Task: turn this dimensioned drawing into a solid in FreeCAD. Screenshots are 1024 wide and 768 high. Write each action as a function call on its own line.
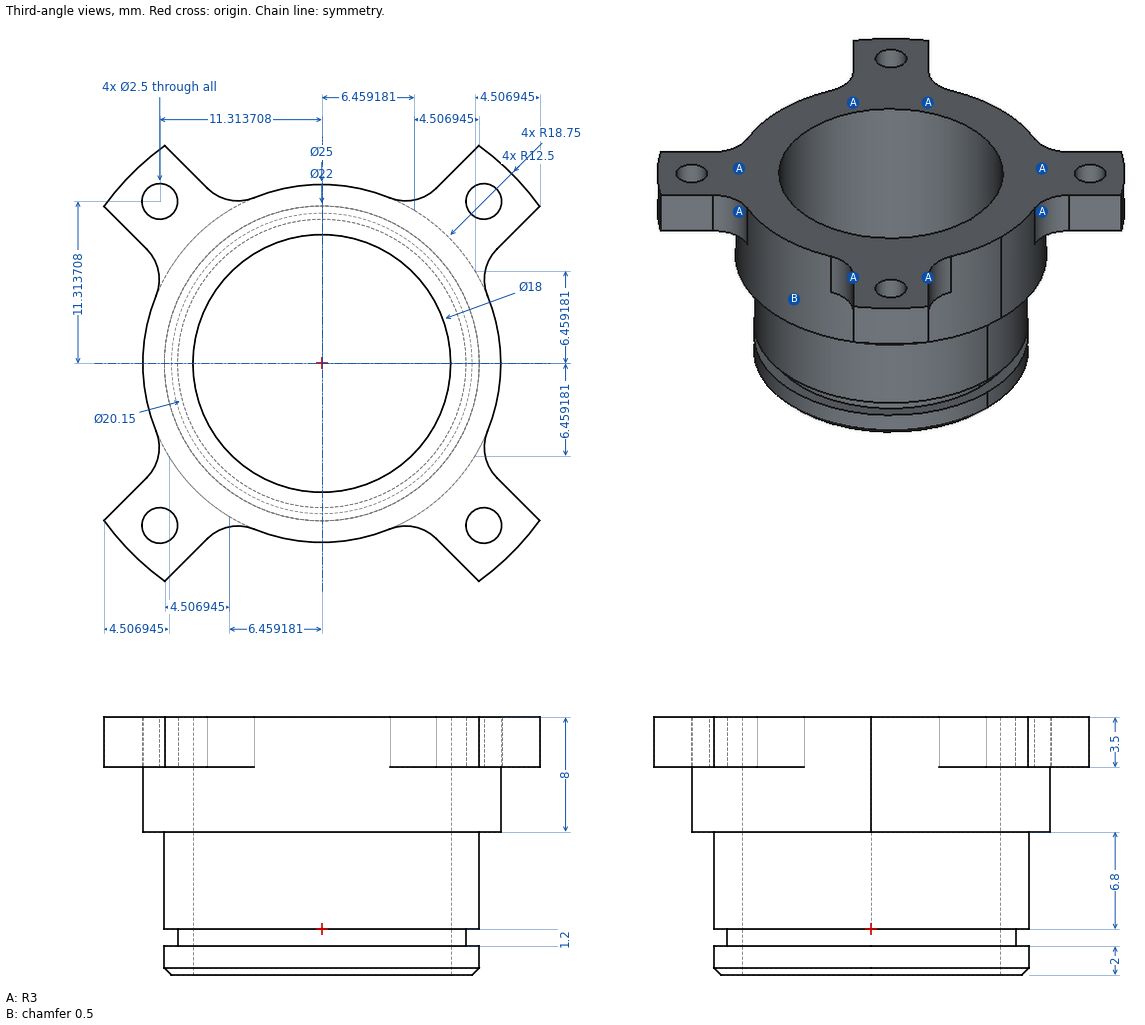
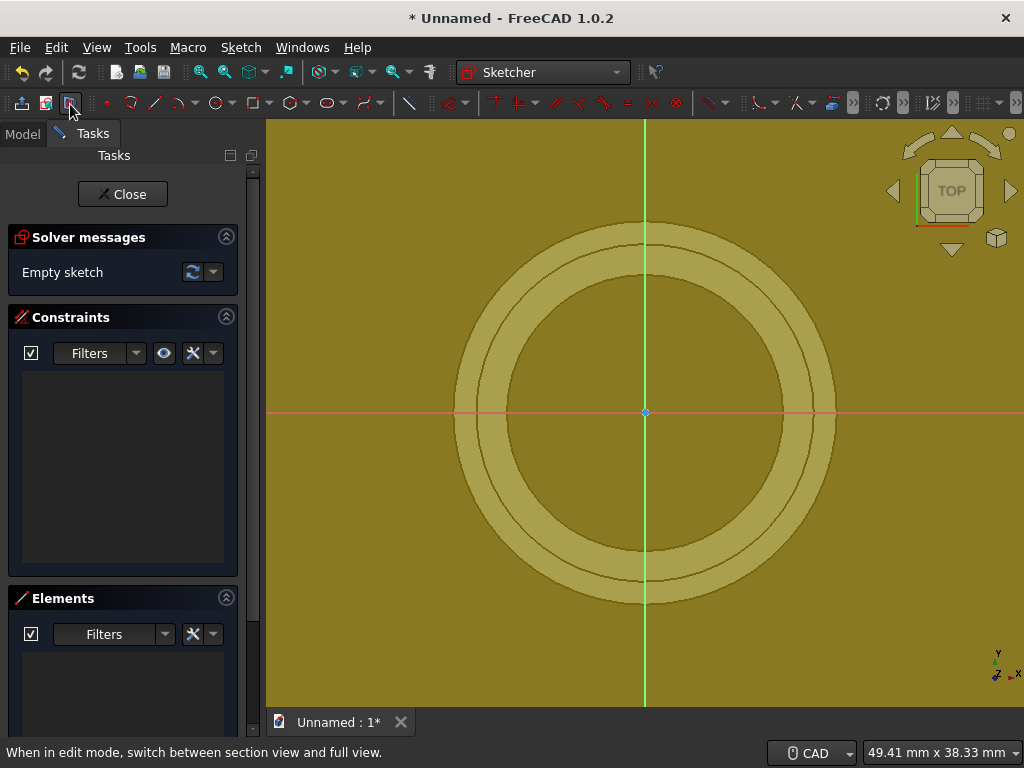
scroll(294, 413, down, 1)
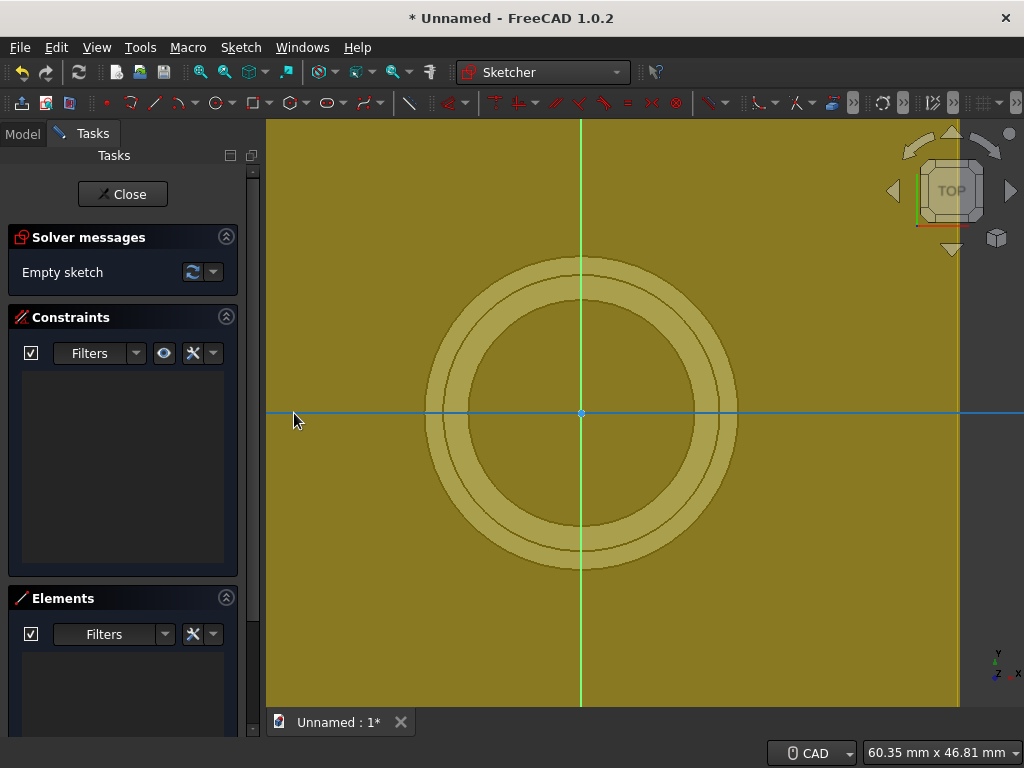
click(156, 104)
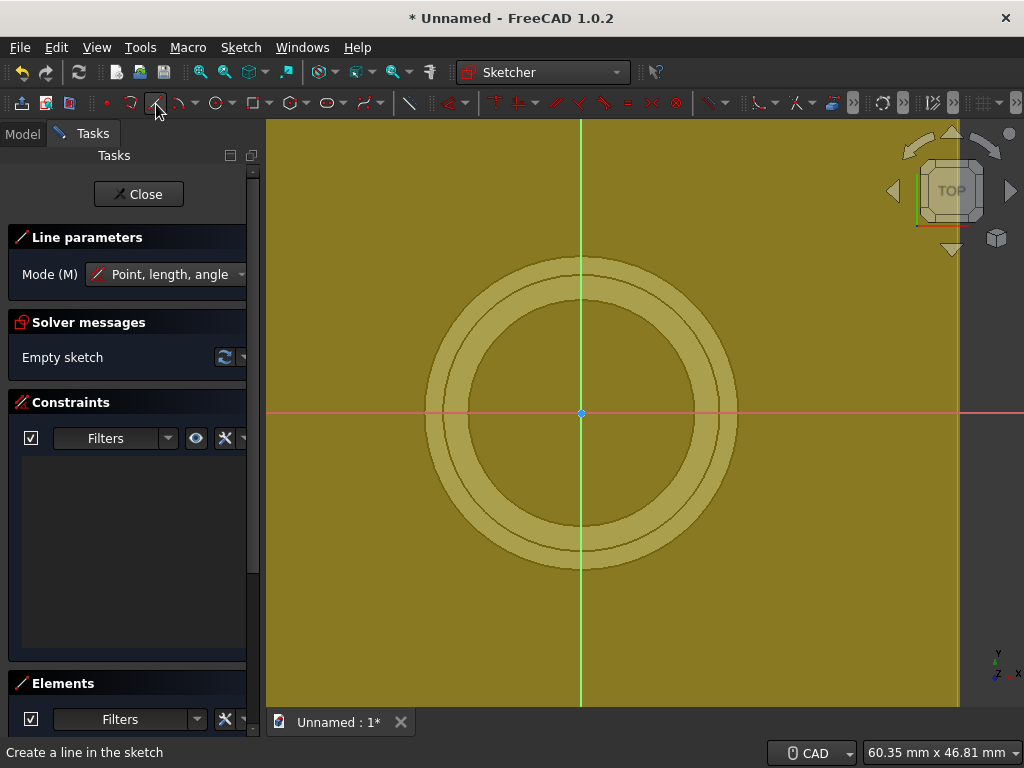
click(719, 222)
click(663, 279)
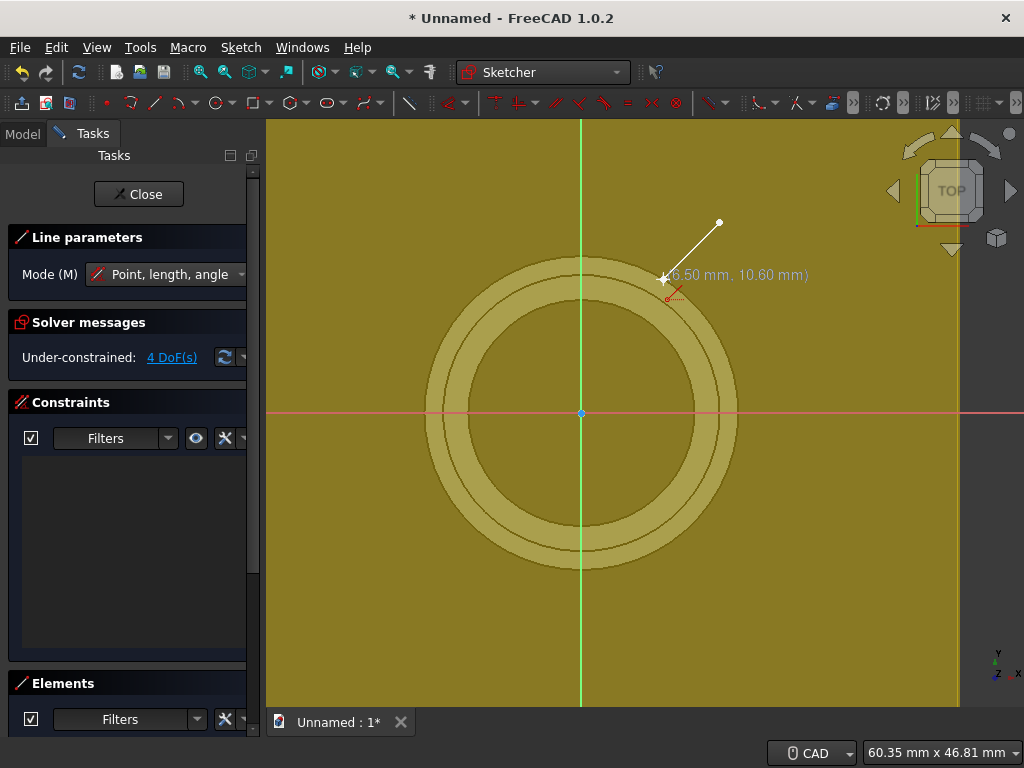
click(716, 332)
click(772, 275)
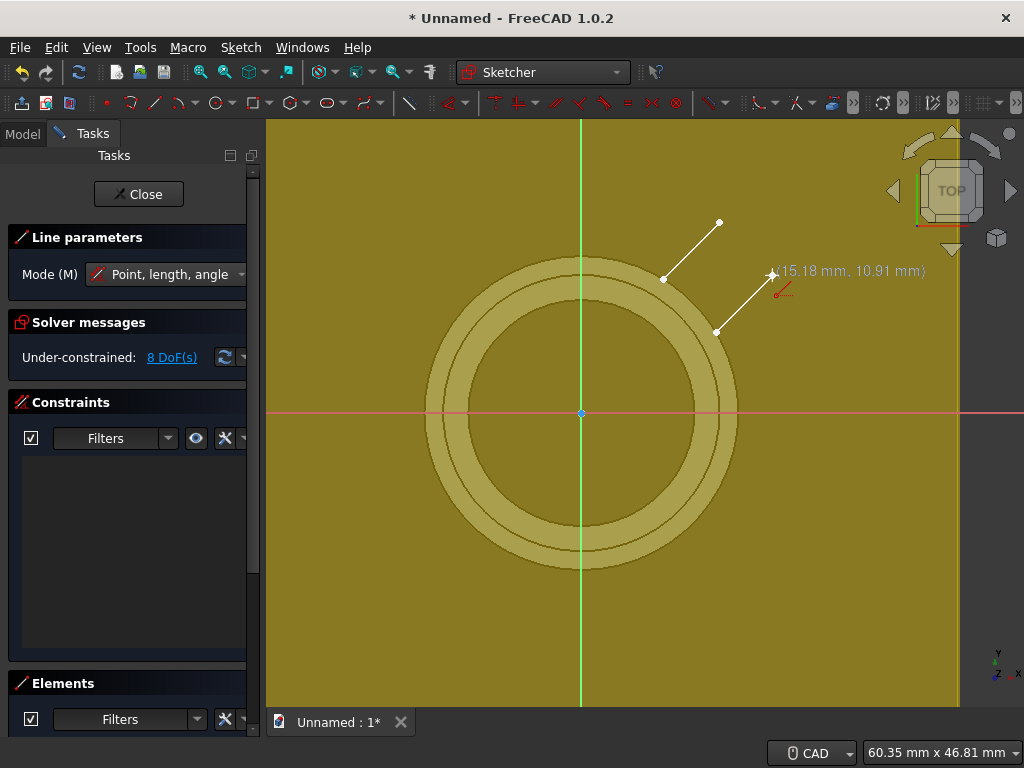
click(198, 104)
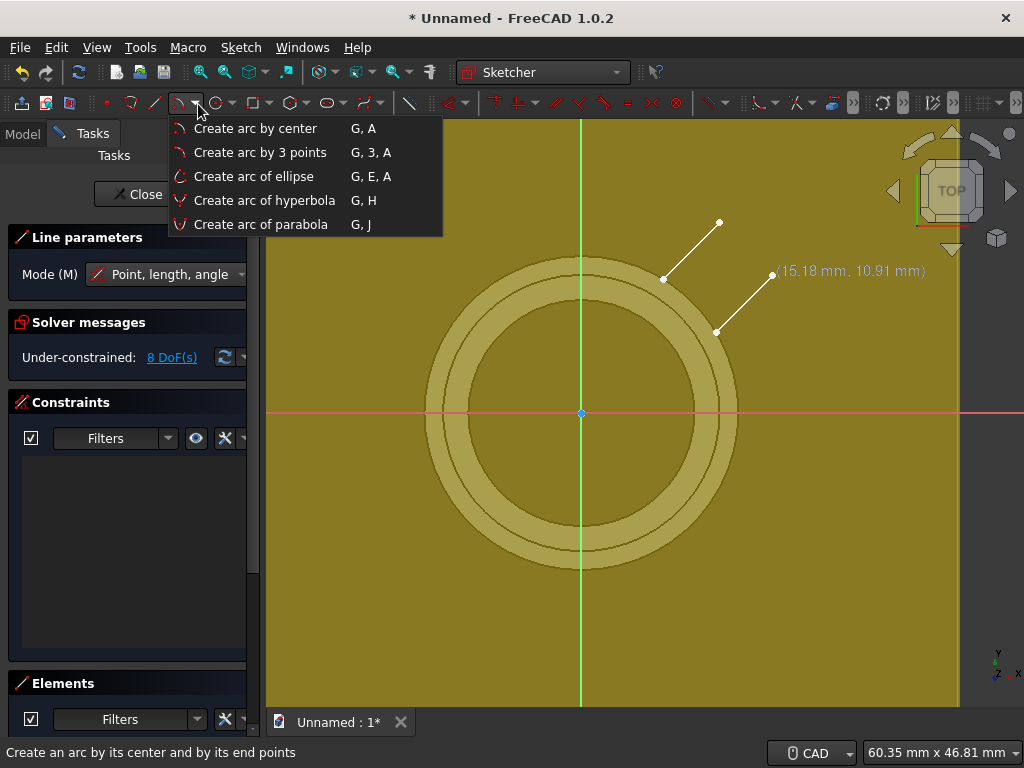
click(306, 152)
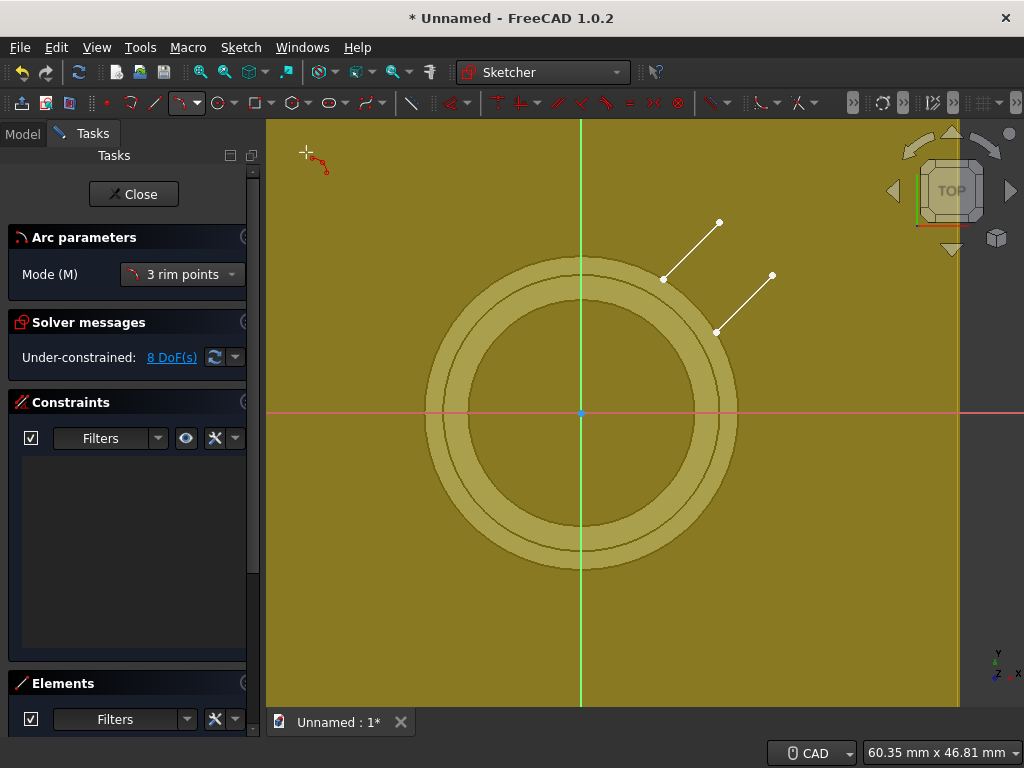
click(663, 280)
click(716, 333)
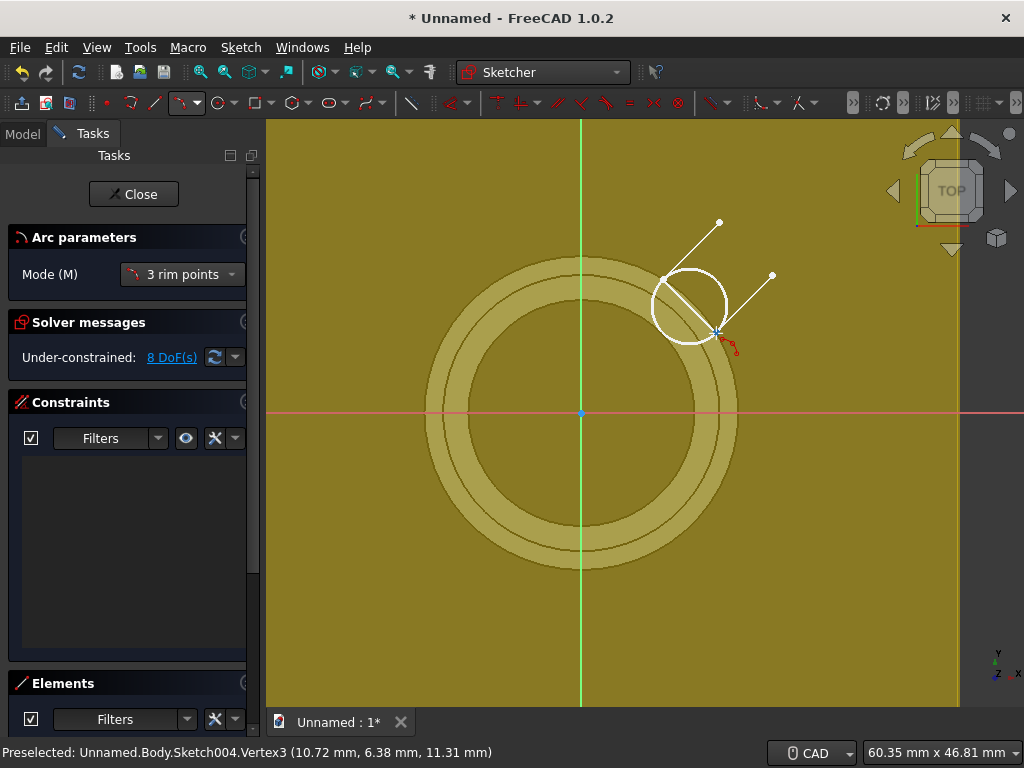
scroll(692, 302, up, 7)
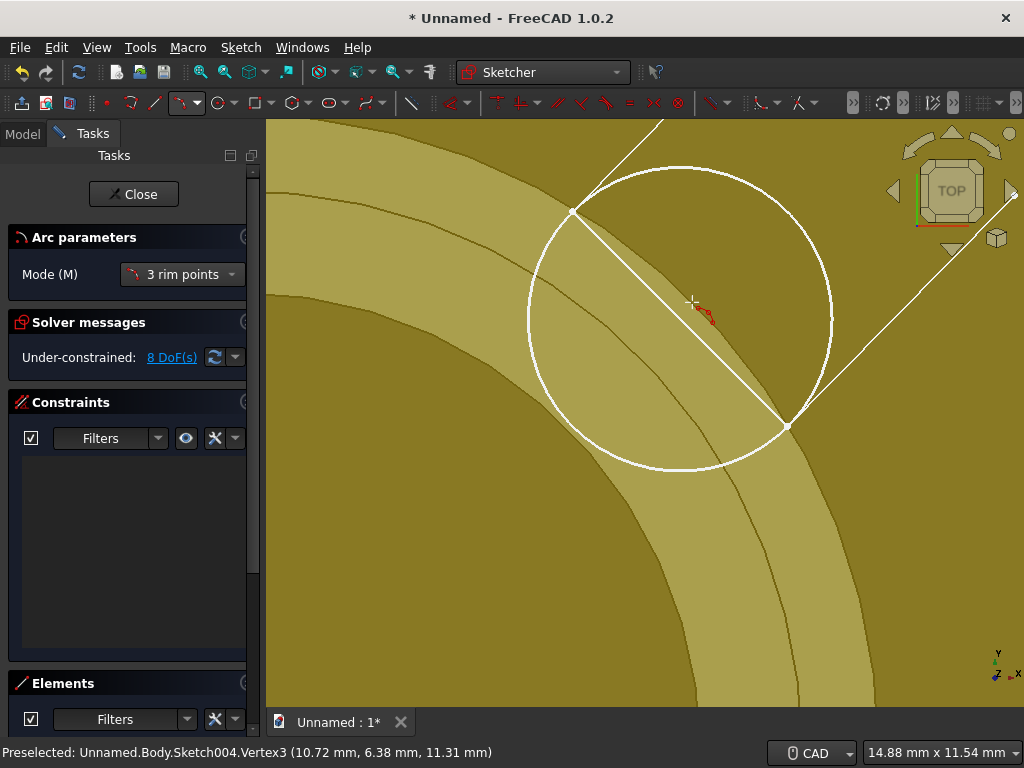
click(692, 301)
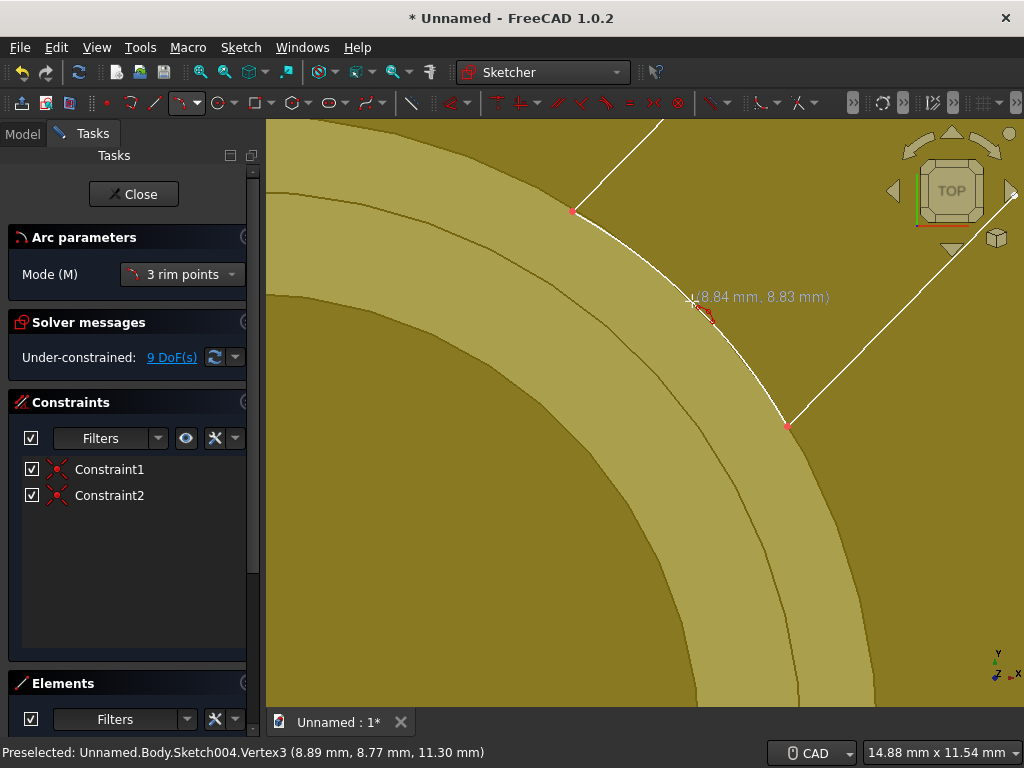
scroll(686, 302, down, 7)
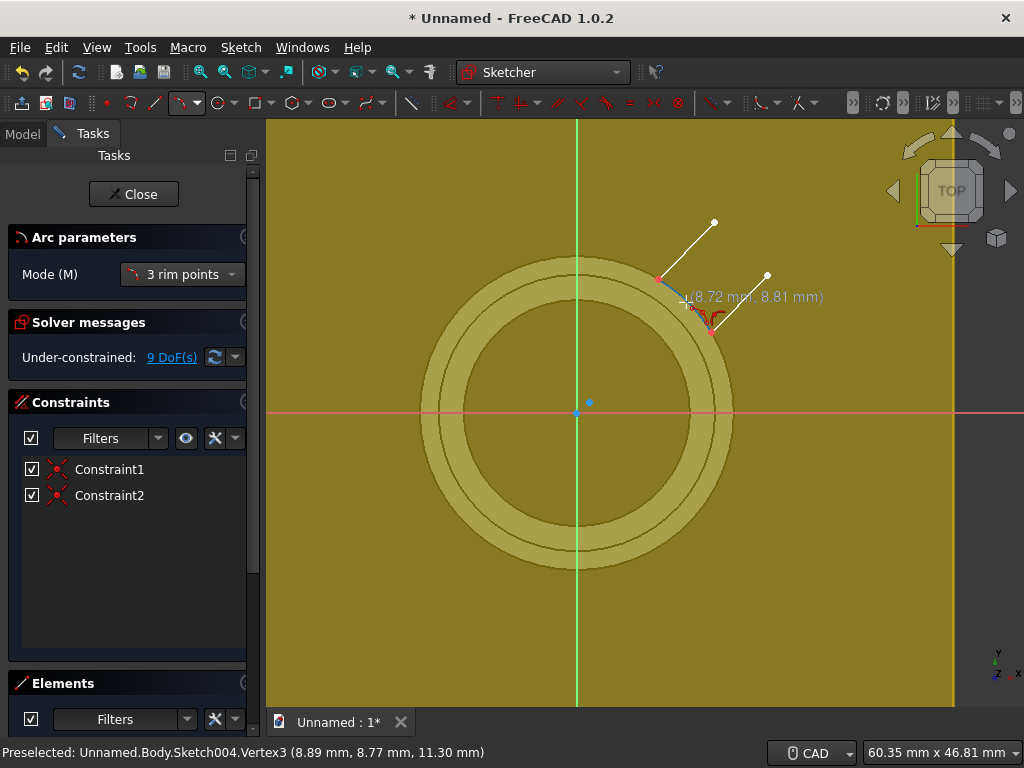
click(767, 276)
click(714, 223)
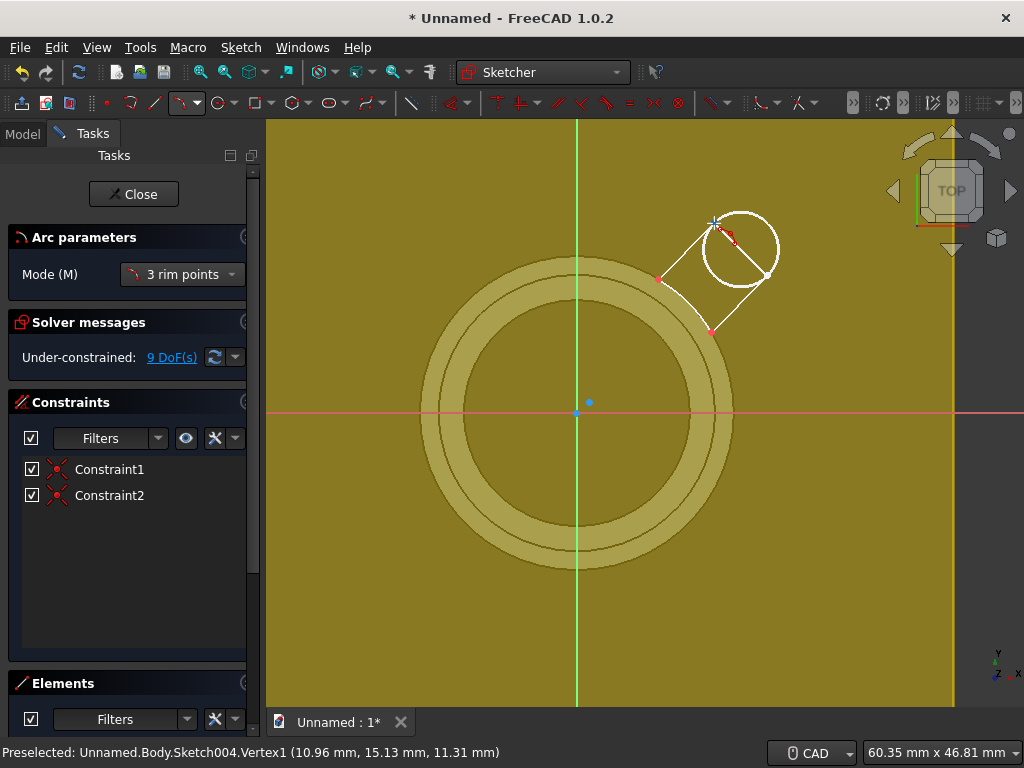
scroll(743, 247, up, 9)